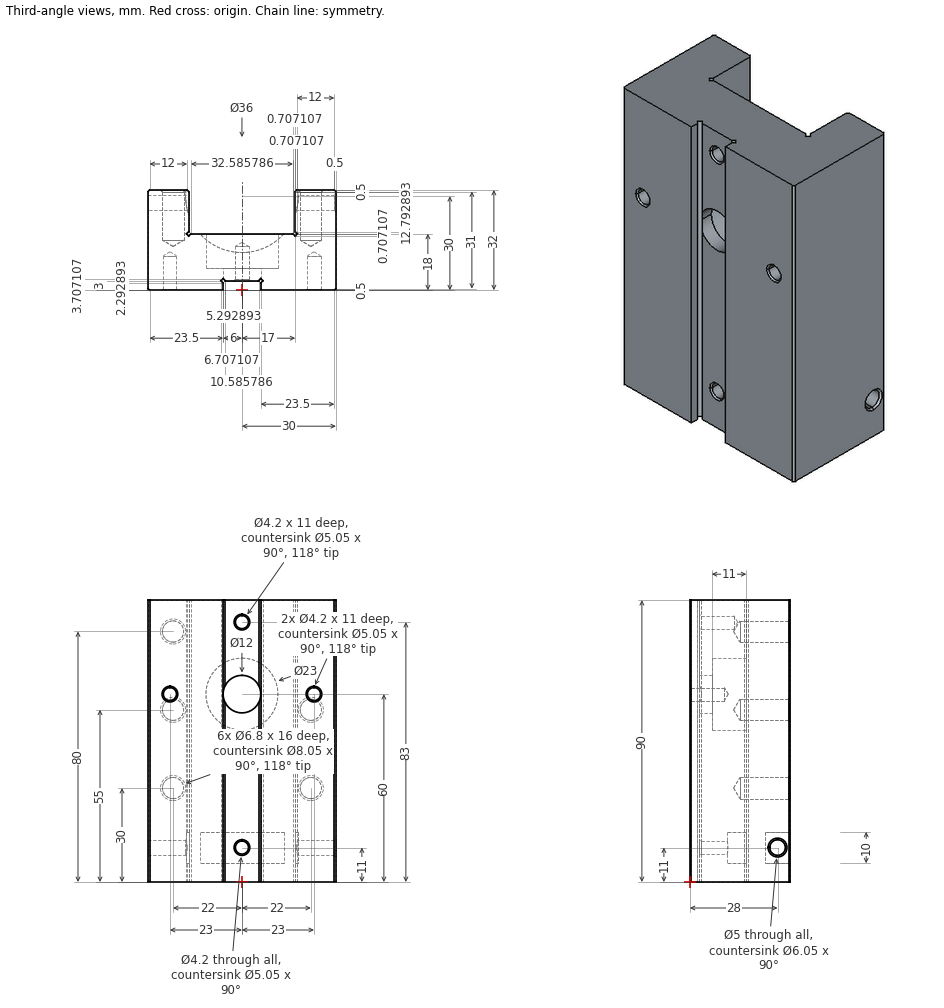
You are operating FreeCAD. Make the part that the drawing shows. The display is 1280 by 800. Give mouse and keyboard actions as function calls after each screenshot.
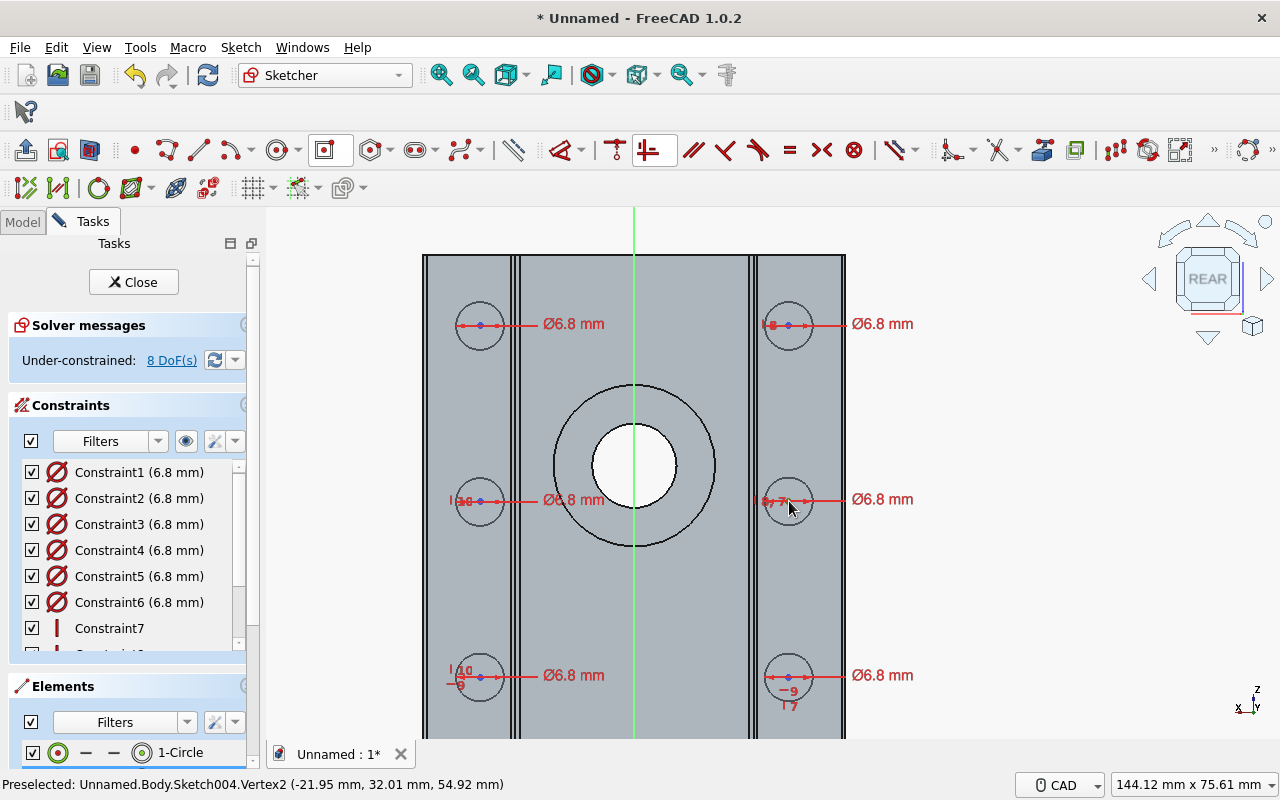
click(480, 502)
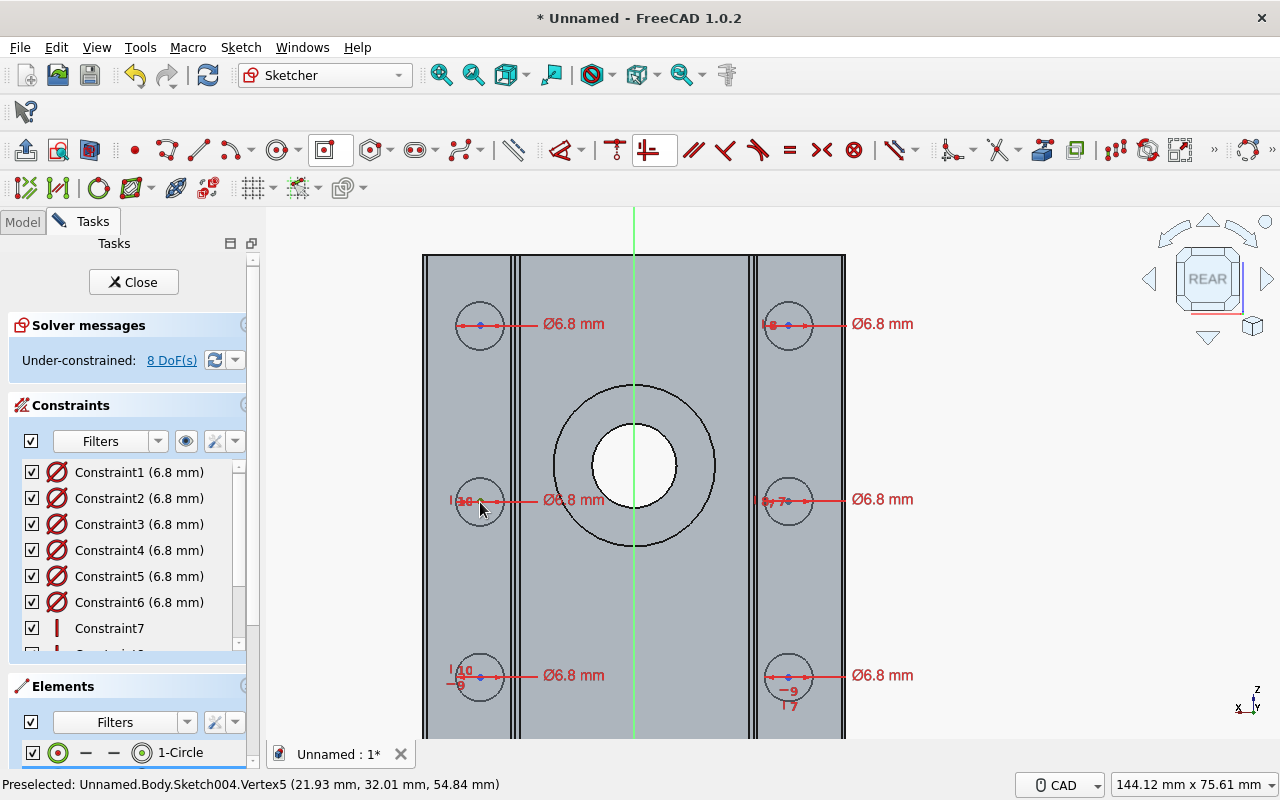
click(672, 150)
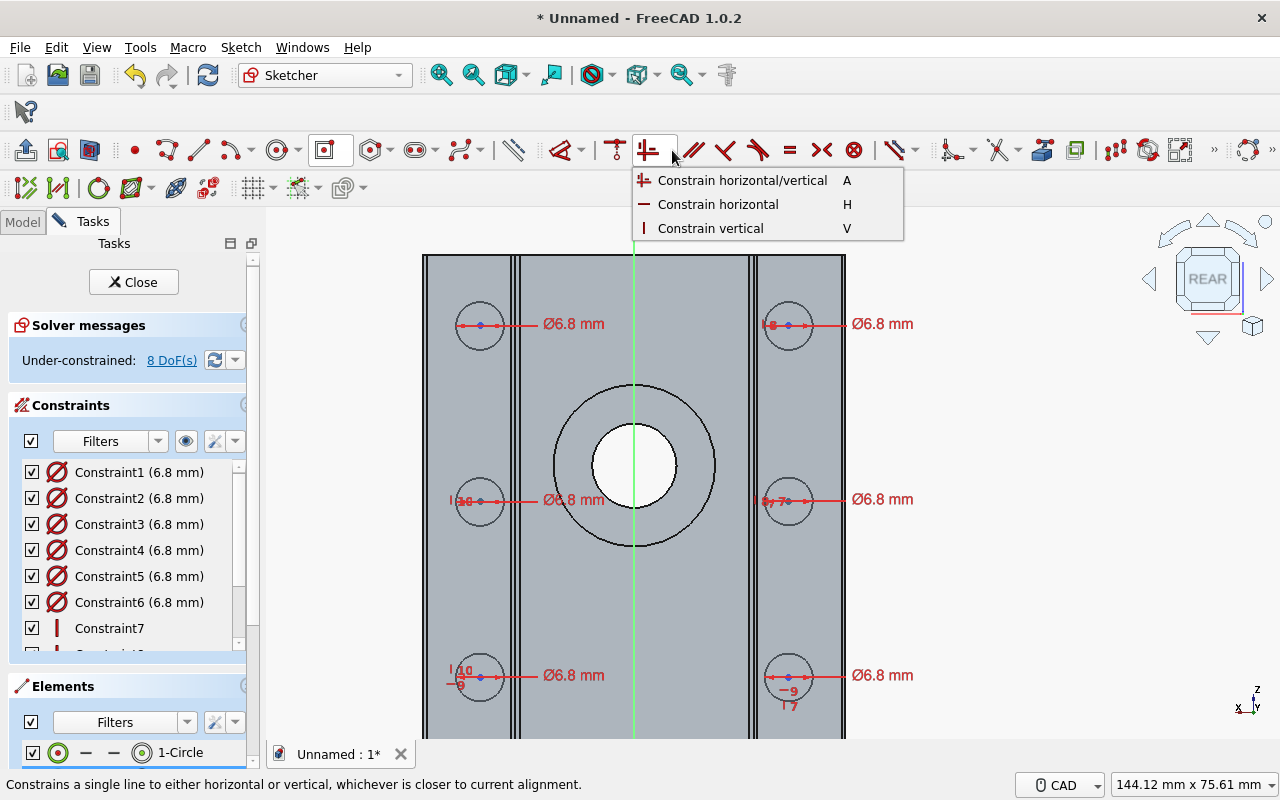
click(768, 204)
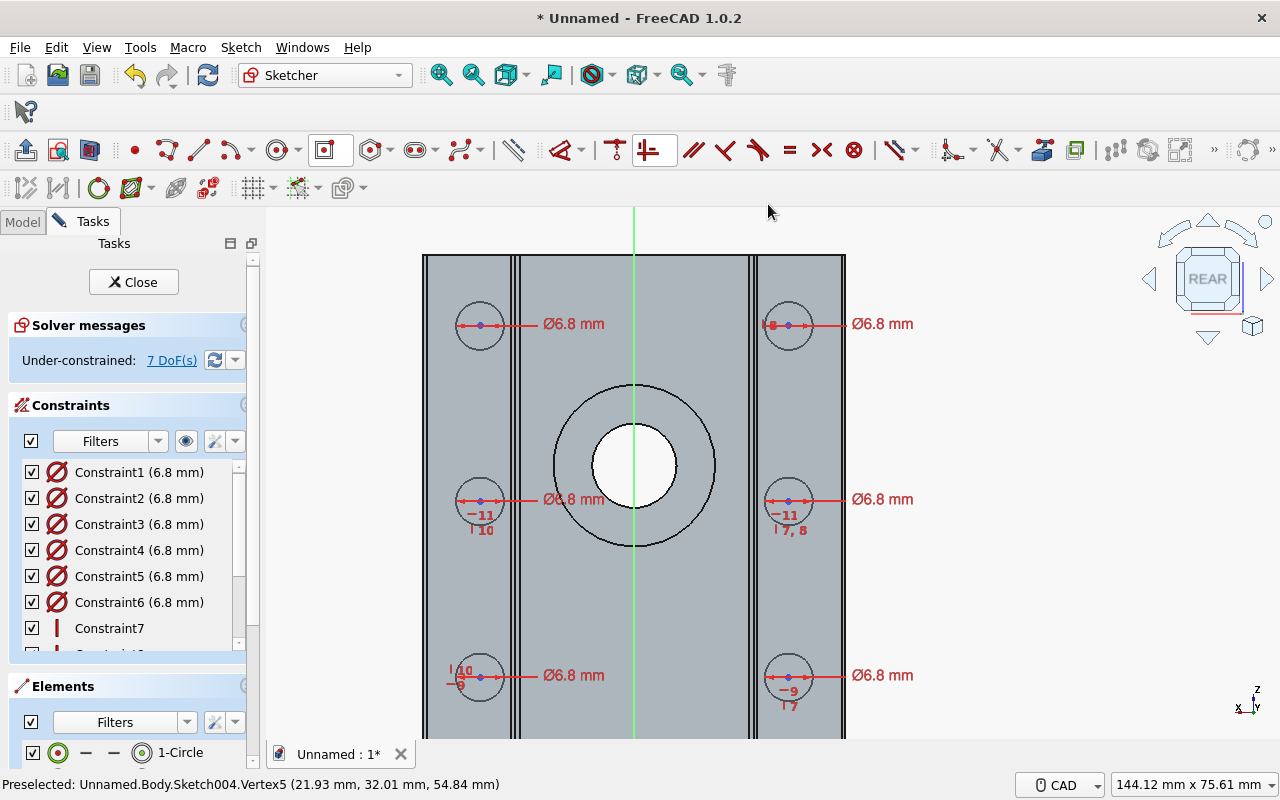
click(480, 501)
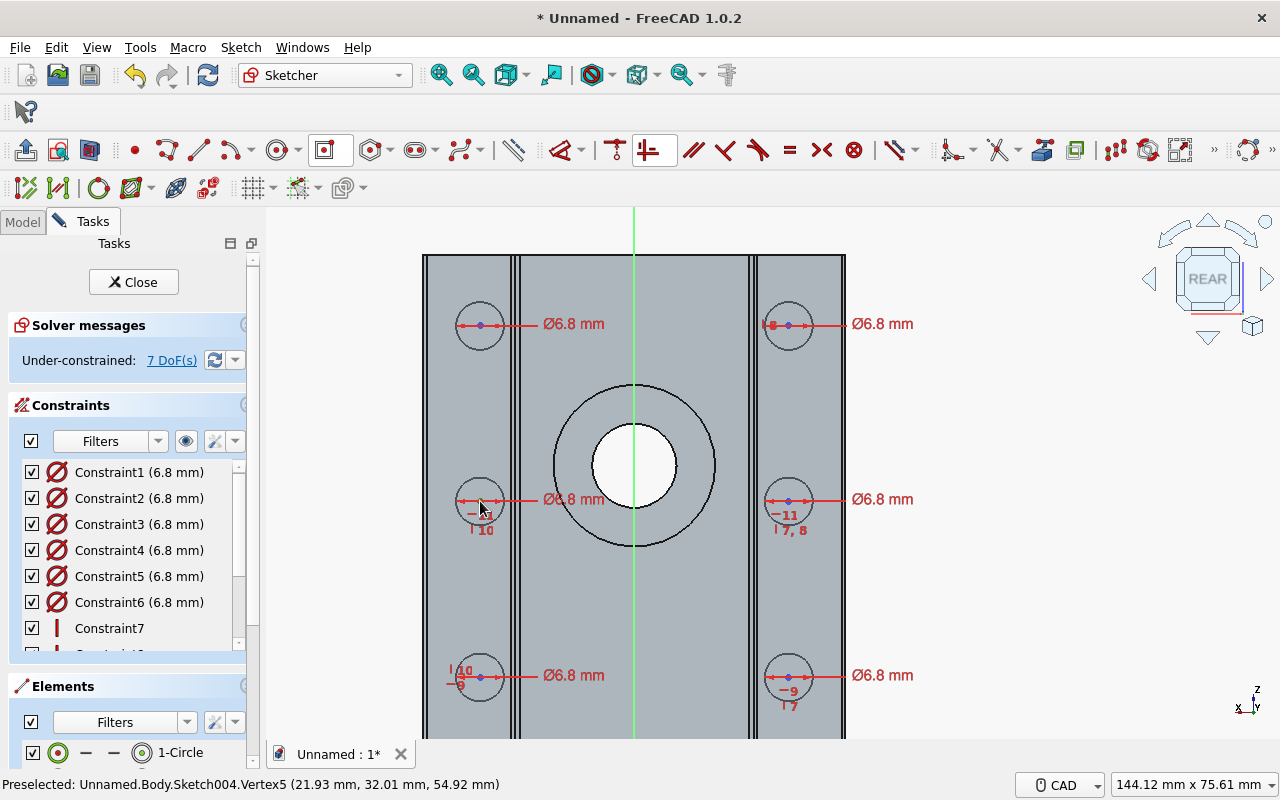
click(480, 326)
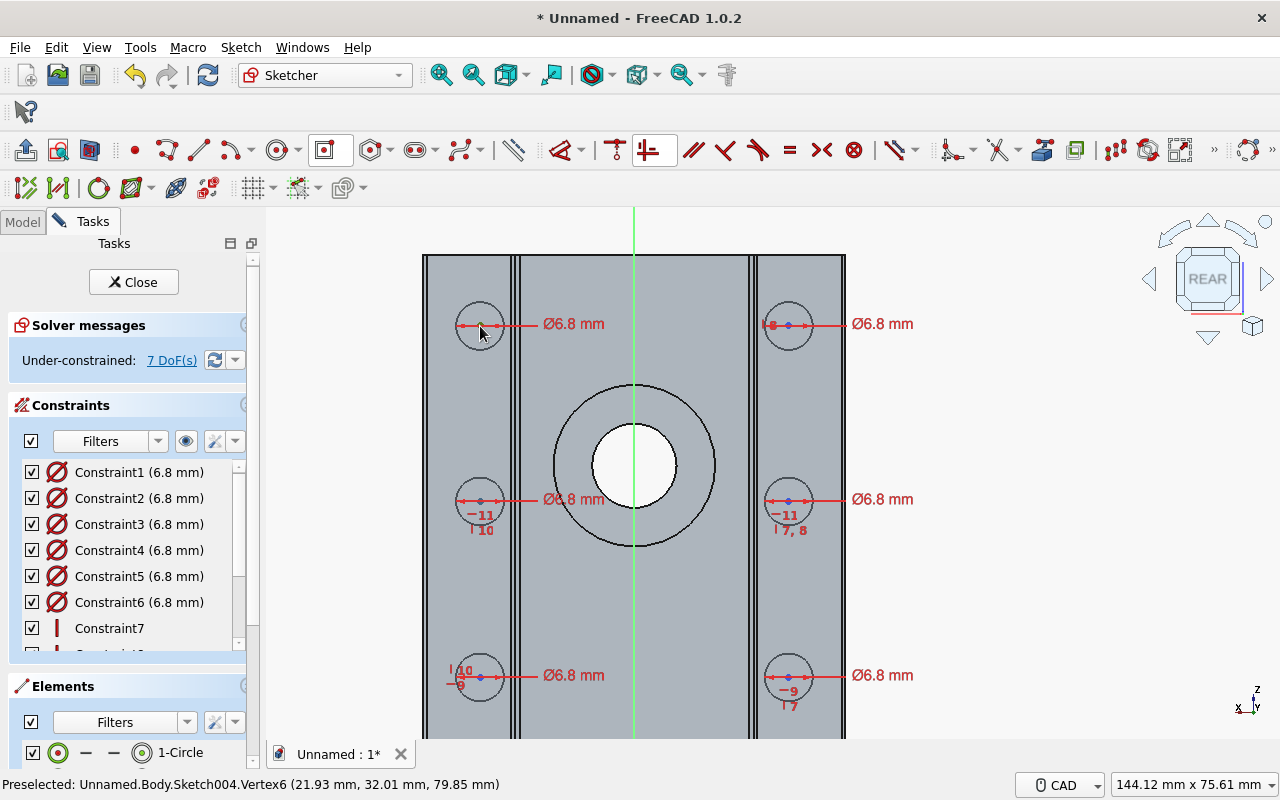
click(672, 150)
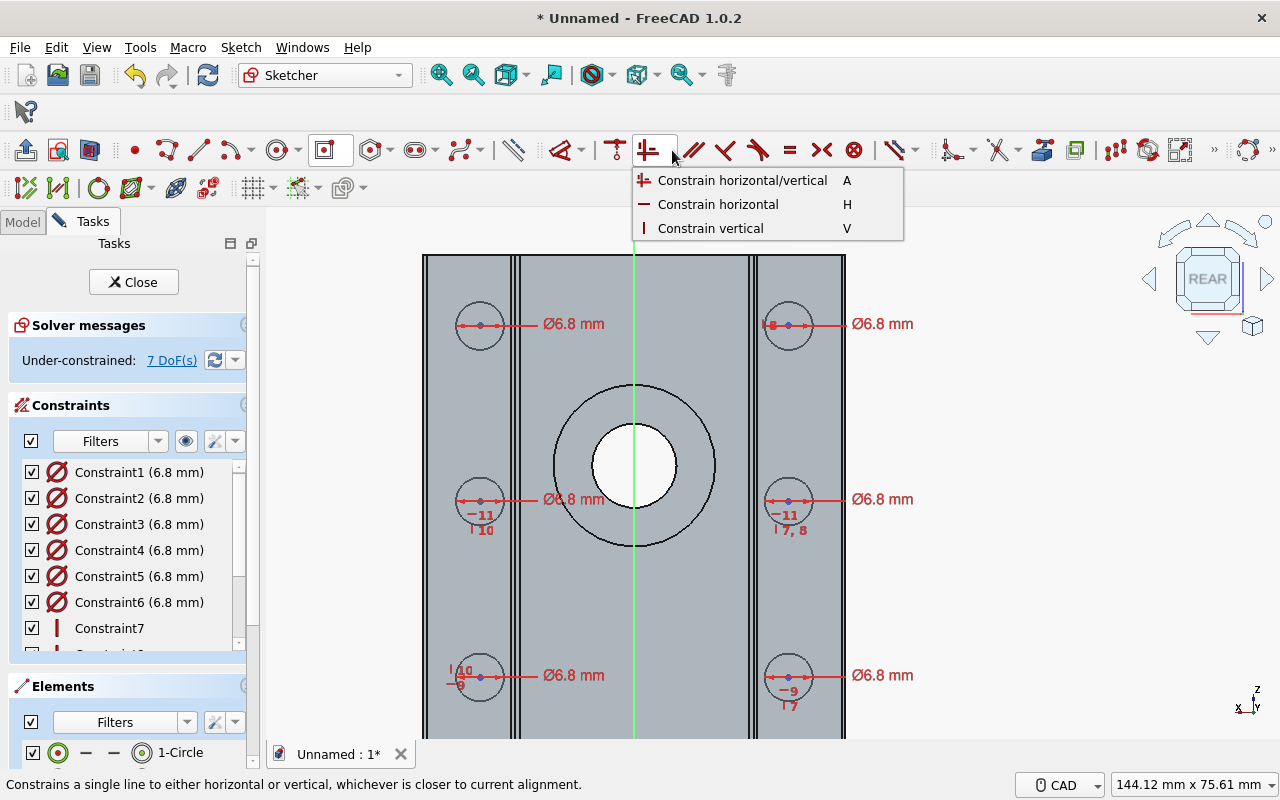
click(768, 228)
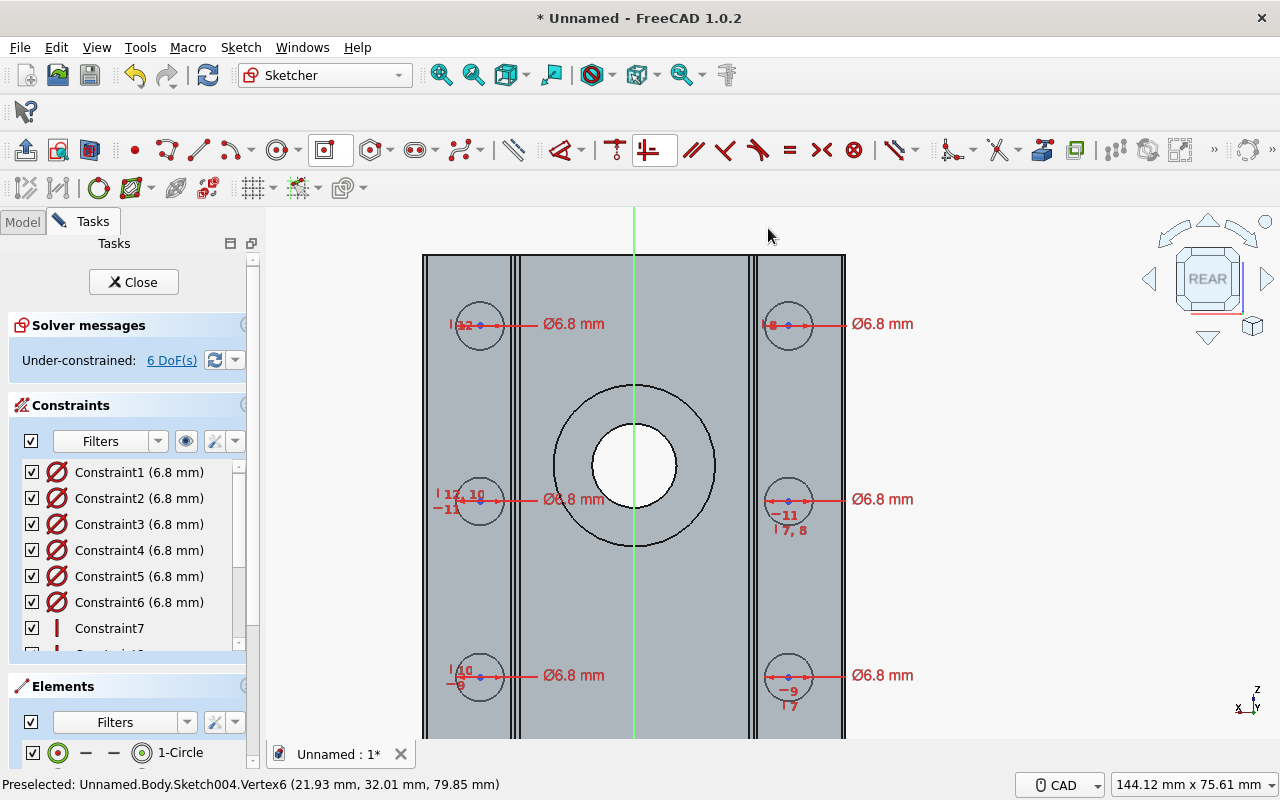
click(789, 326)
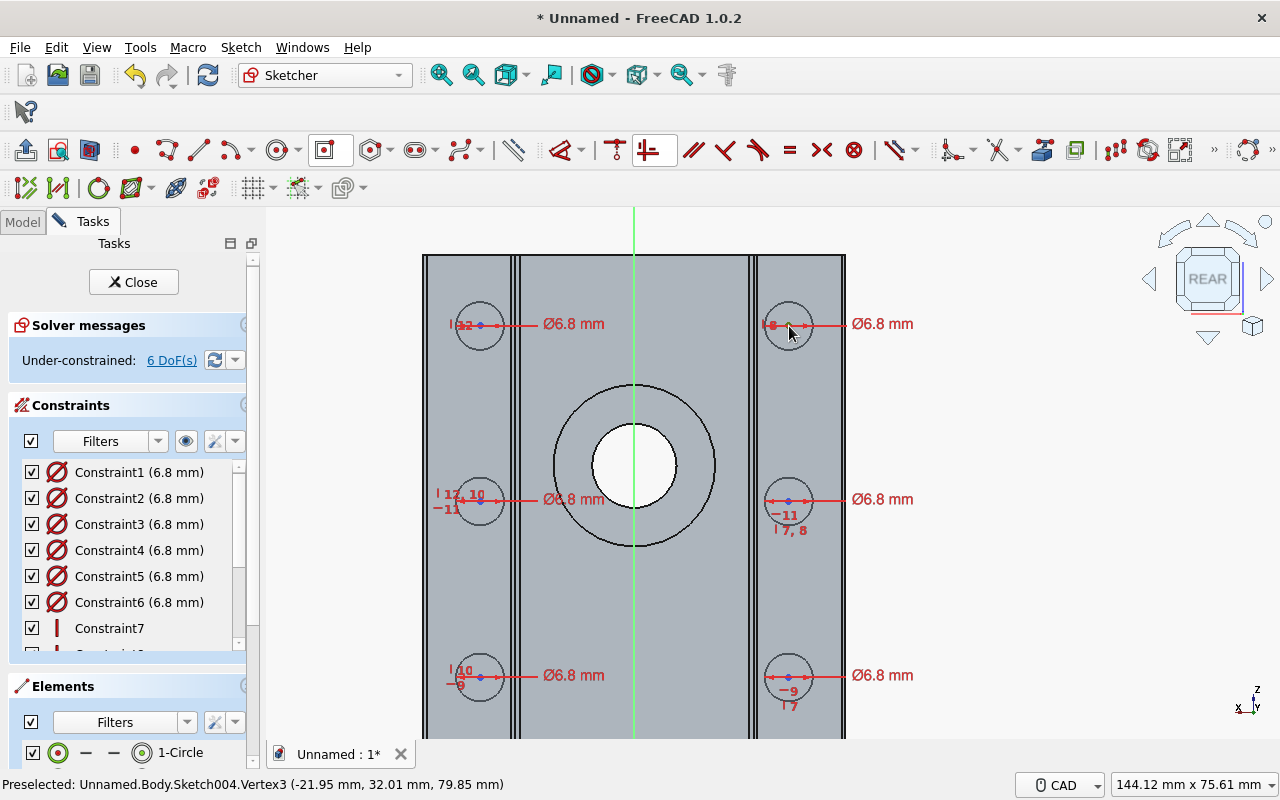
click(480, 326)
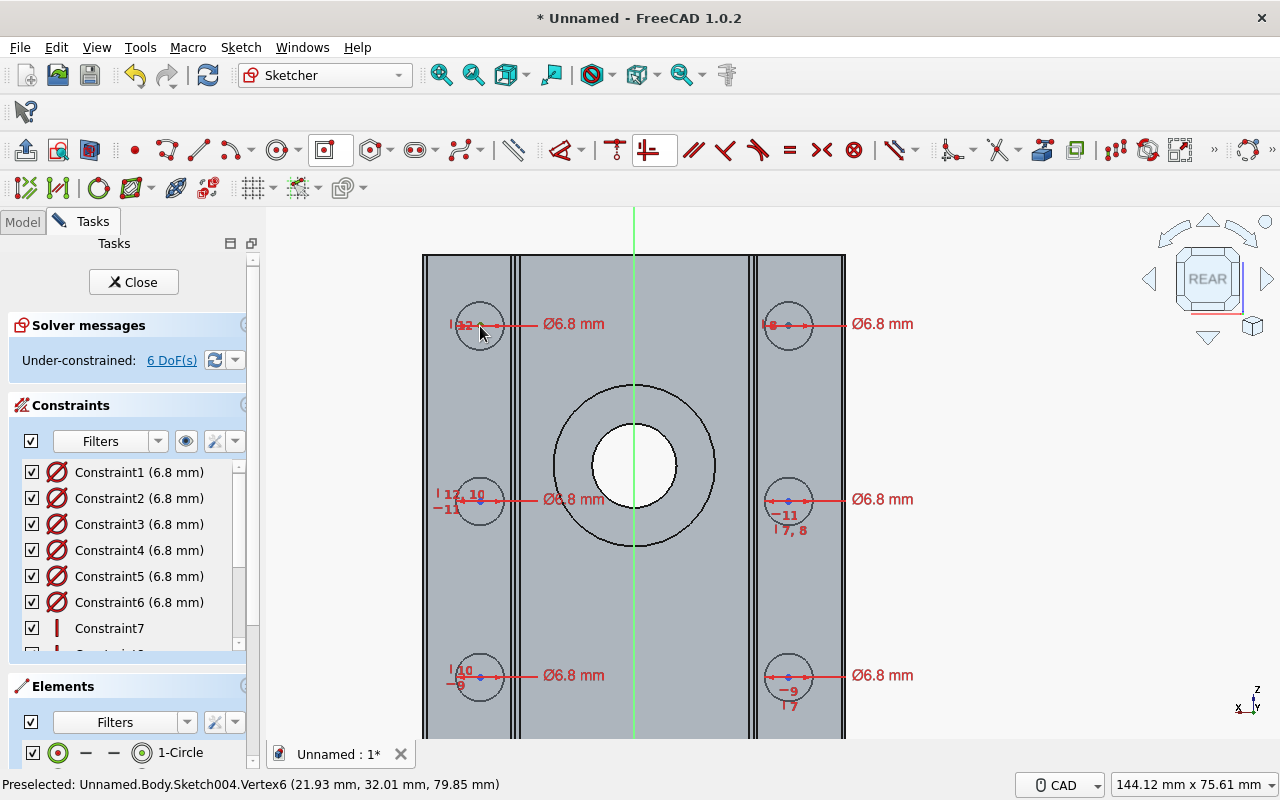
key(h)